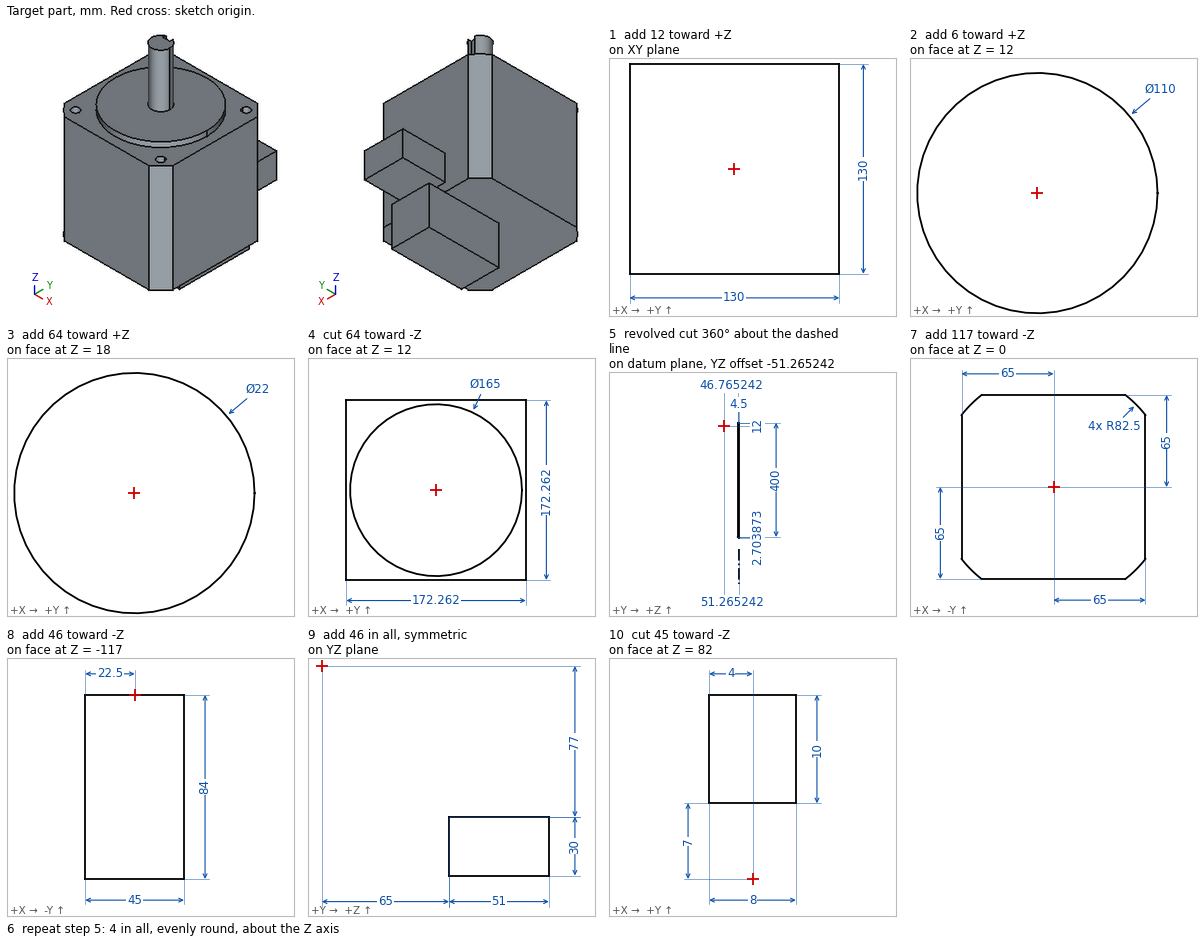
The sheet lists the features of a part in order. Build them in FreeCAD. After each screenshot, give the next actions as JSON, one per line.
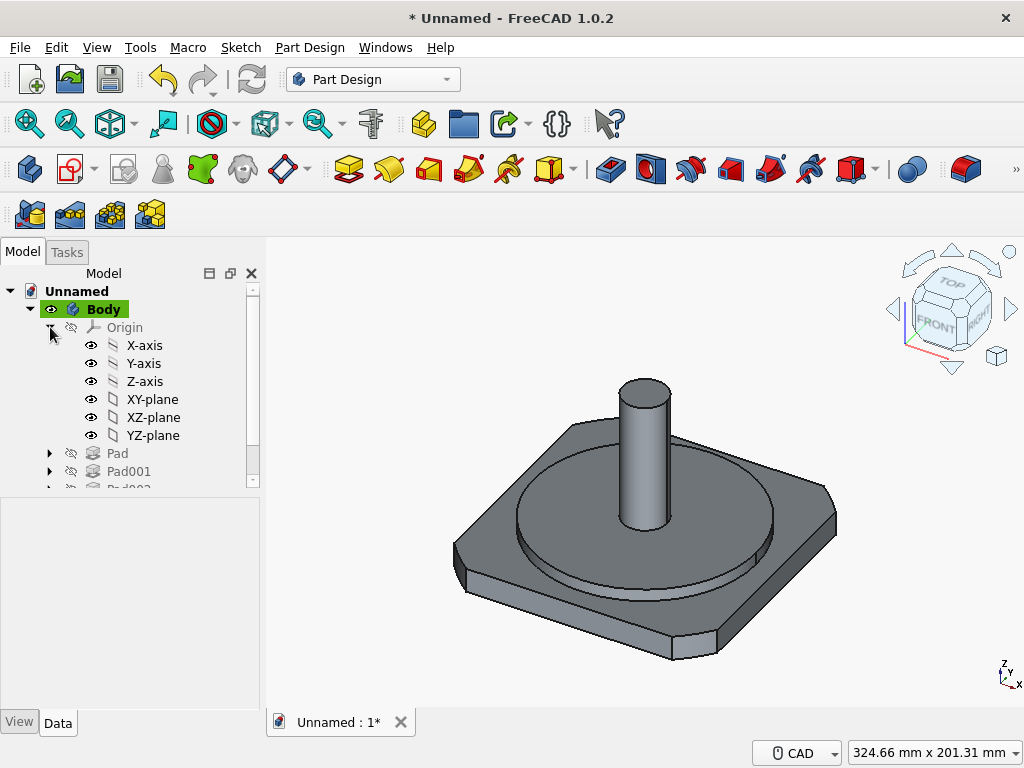
{"action": "left_click", "coordinate": [136, 435]}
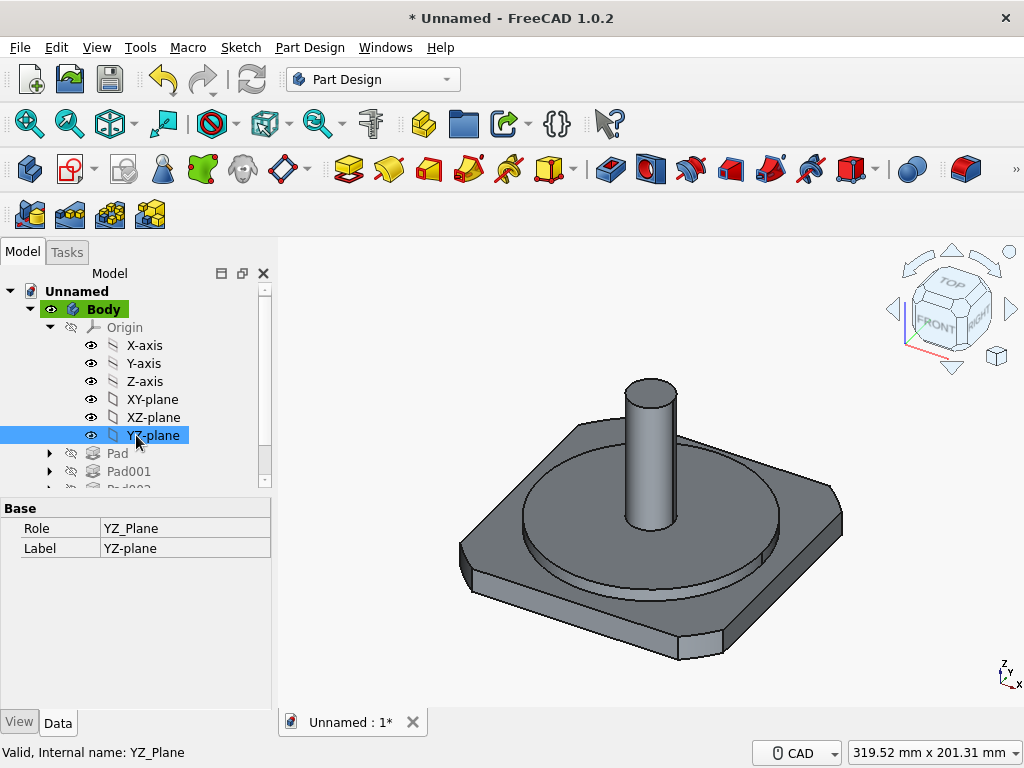
{"action": "left_click", "coordinate": [284, 170]}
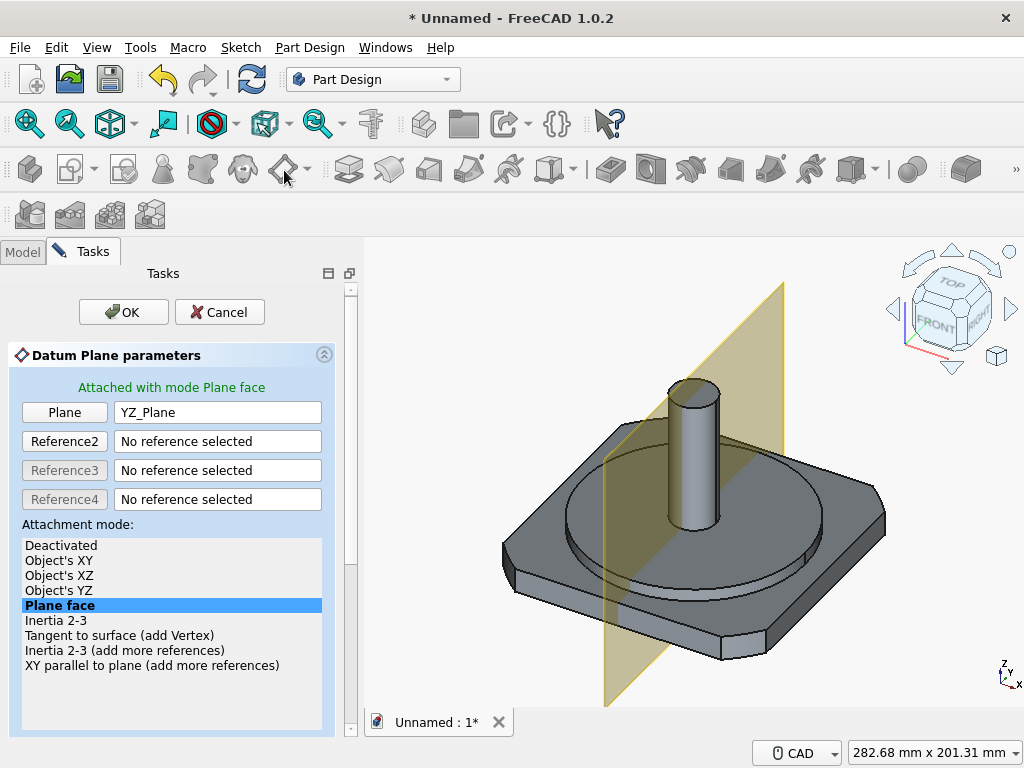
{"action": "scroll", "coordinate": [351, 510], "scroll_direction": "down", "scroll_amount": 3}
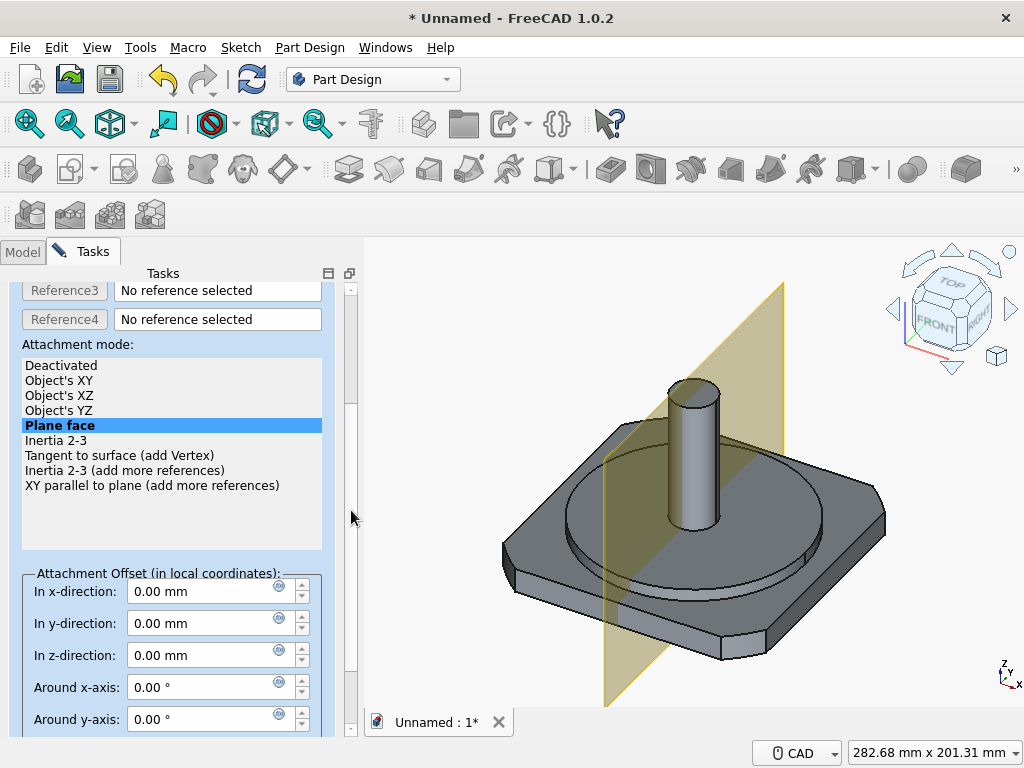
{"action": "triple_click", "coordinate": [210, 655]}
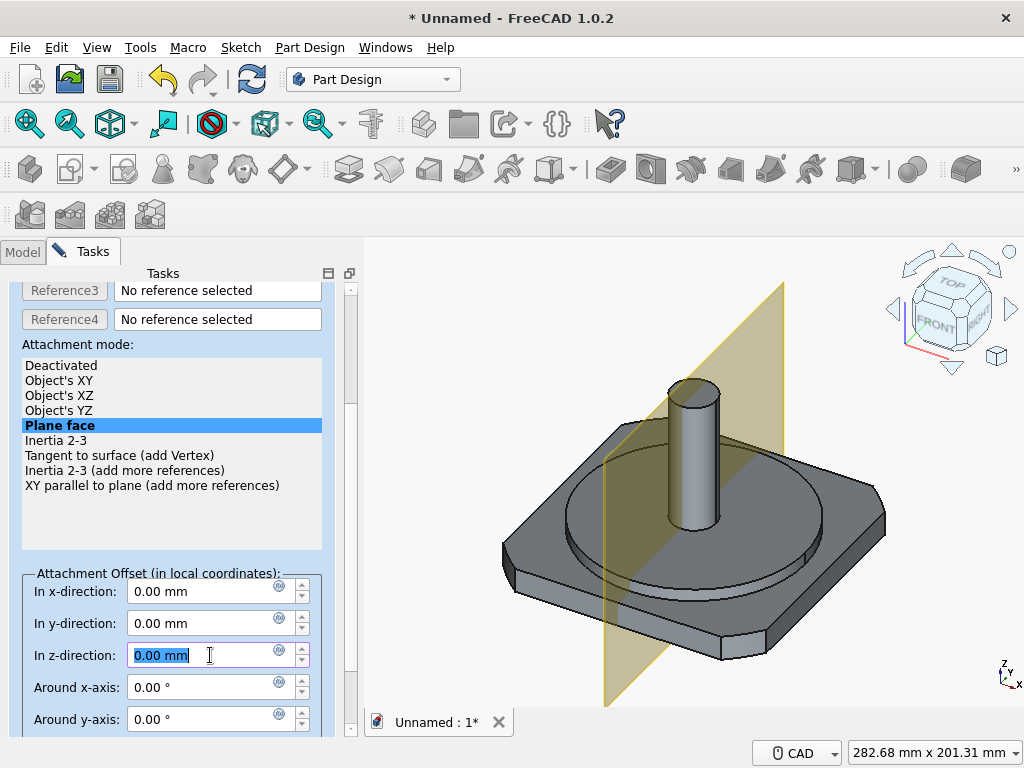
{"action": "type", "text": "-51.265242"}
{"action": "key", "text": "Tab"}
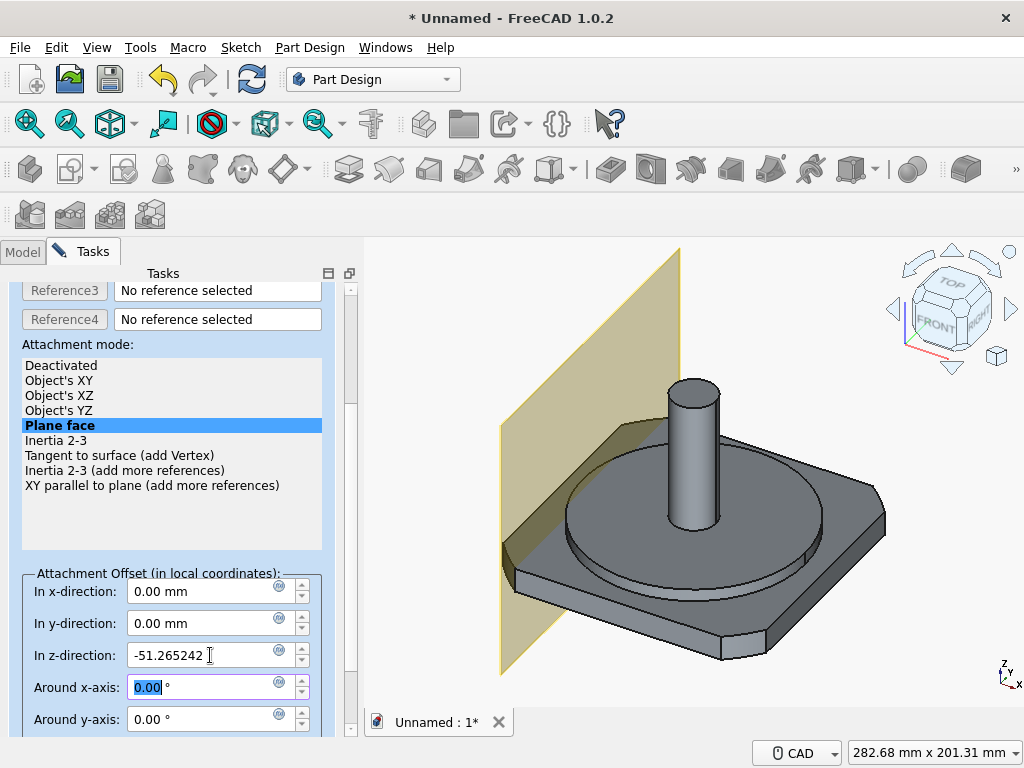
{"action": "scroll", "coordinate": [351, 510], "scroll_direction": "up", "scroll_amount": 4}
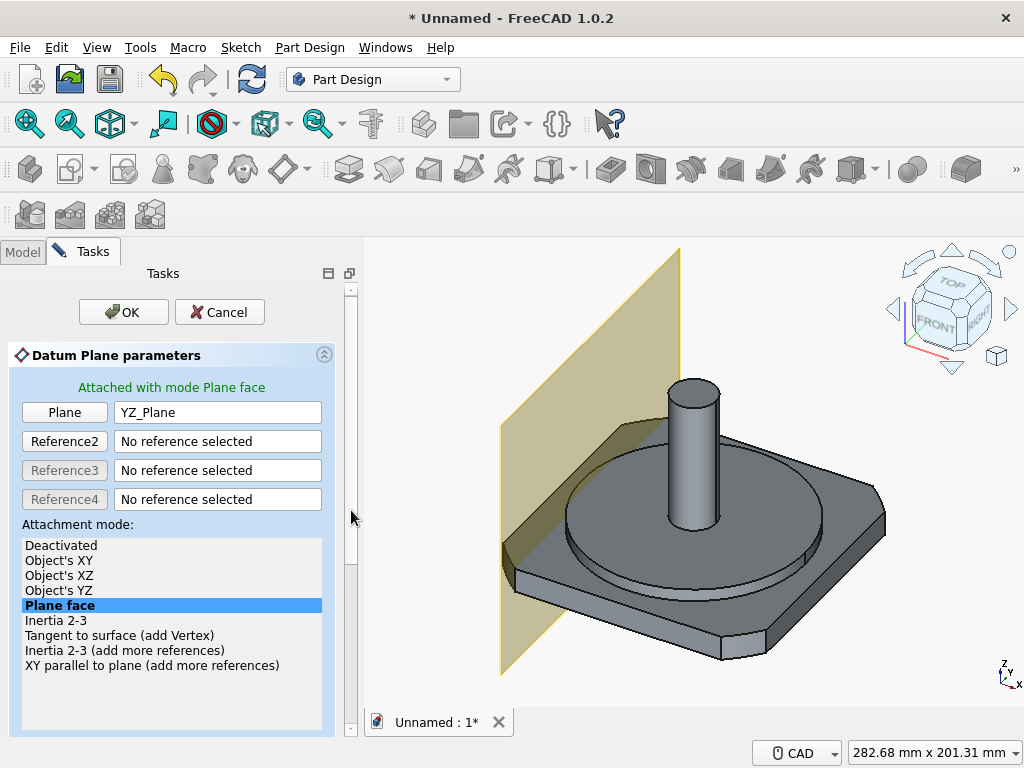
{"action": "left_click", "coordinate": [124, 312]}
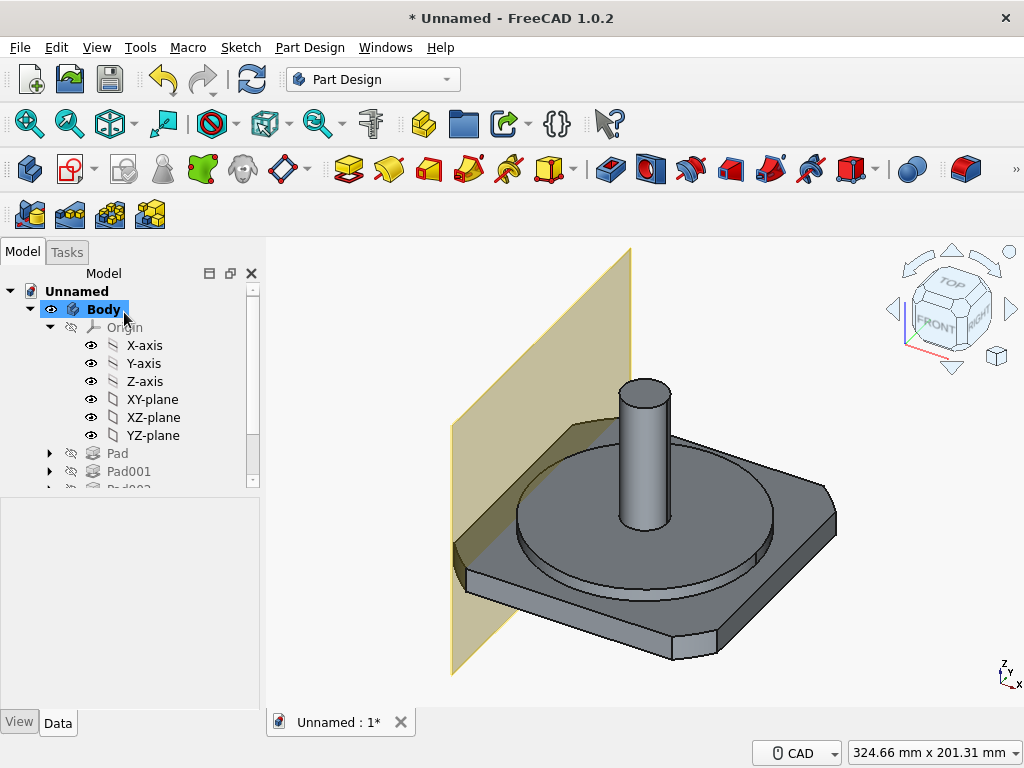
{"action": "scroll", "coordinate": [100, 377], "scroll_direction": "down", "scroll_amount": 3}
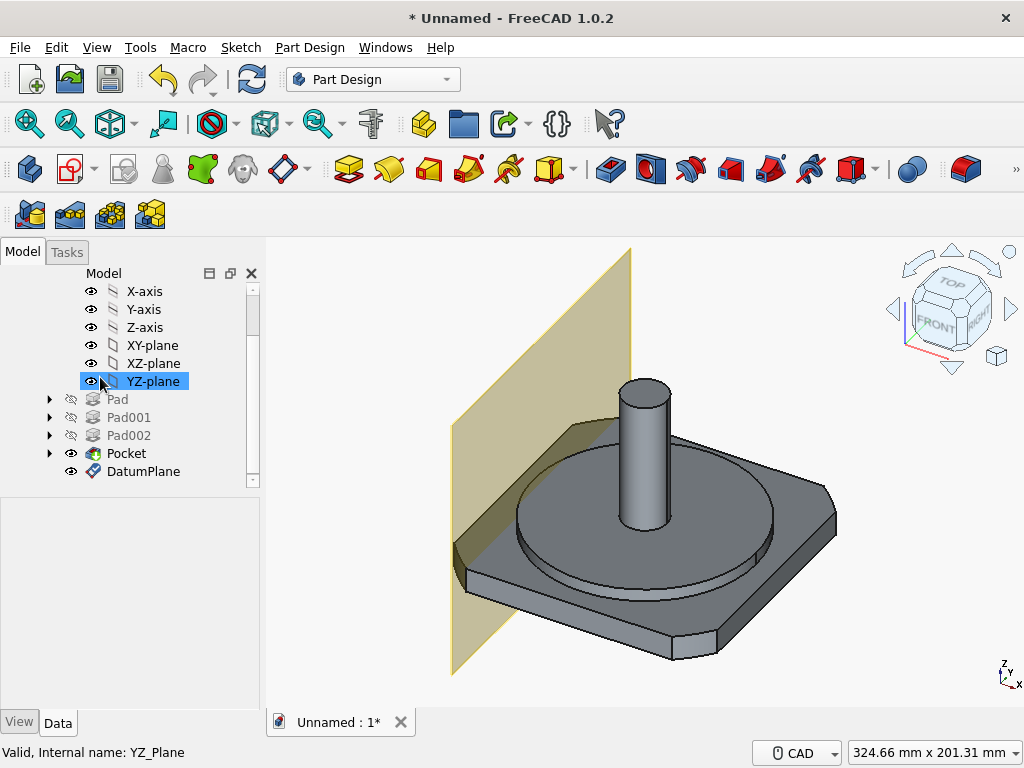
{"action": "left_click", "coordinate": [116, 471]}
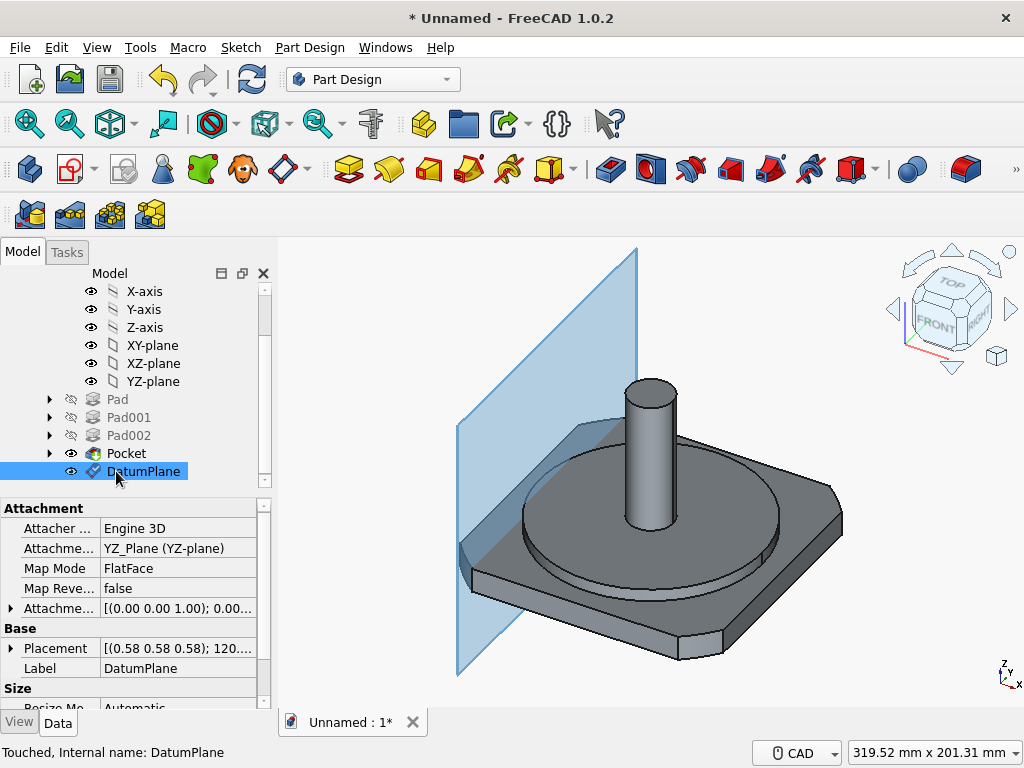
{"action": "left_click", "coordinate": [70, 170]}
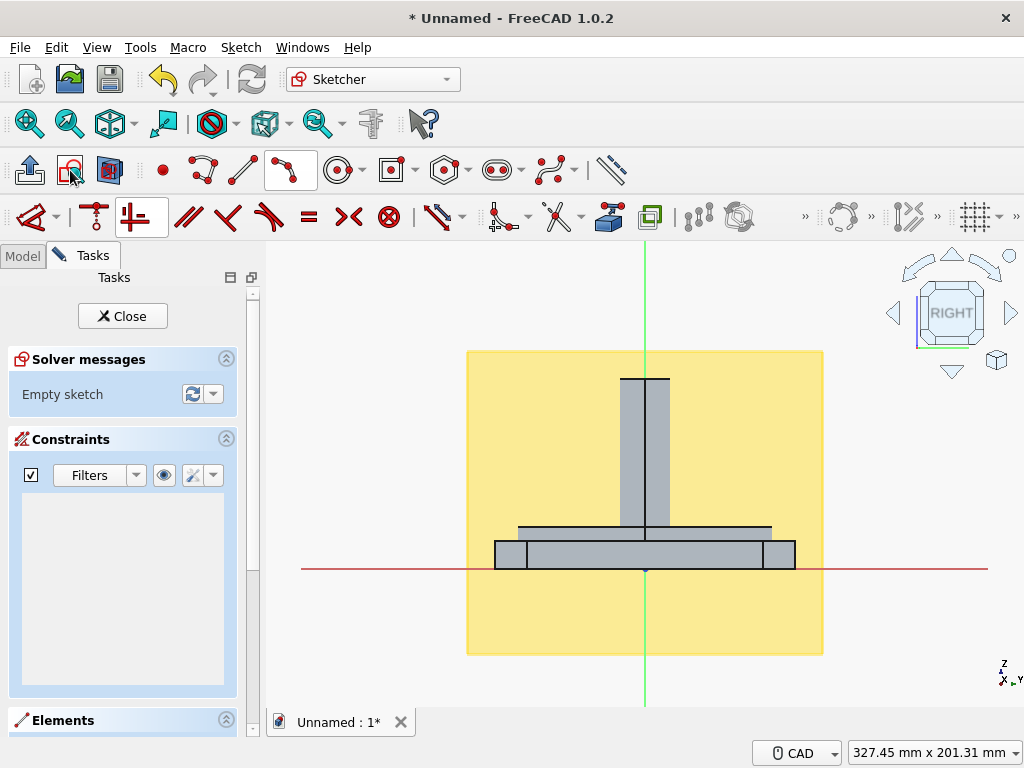
{"action": "left_click", "coordinate": [110, 170]}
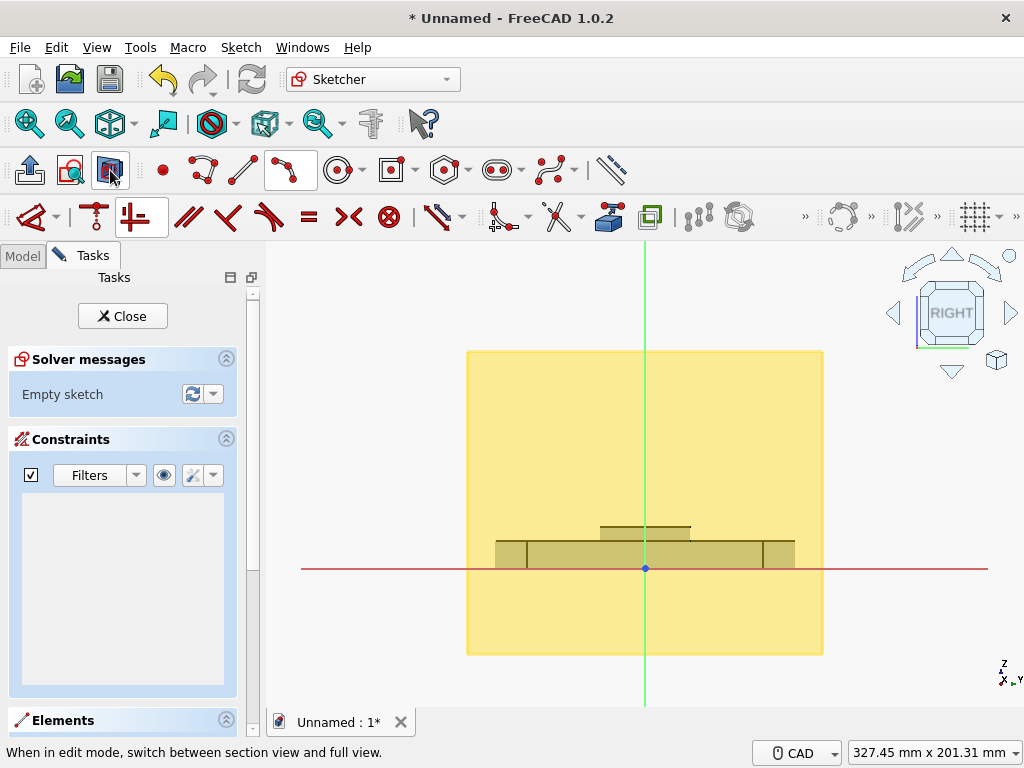
{"action": "scroll", "coordinate": [544, 292], "scroll_direction": "down", "scroll_amount": 8}